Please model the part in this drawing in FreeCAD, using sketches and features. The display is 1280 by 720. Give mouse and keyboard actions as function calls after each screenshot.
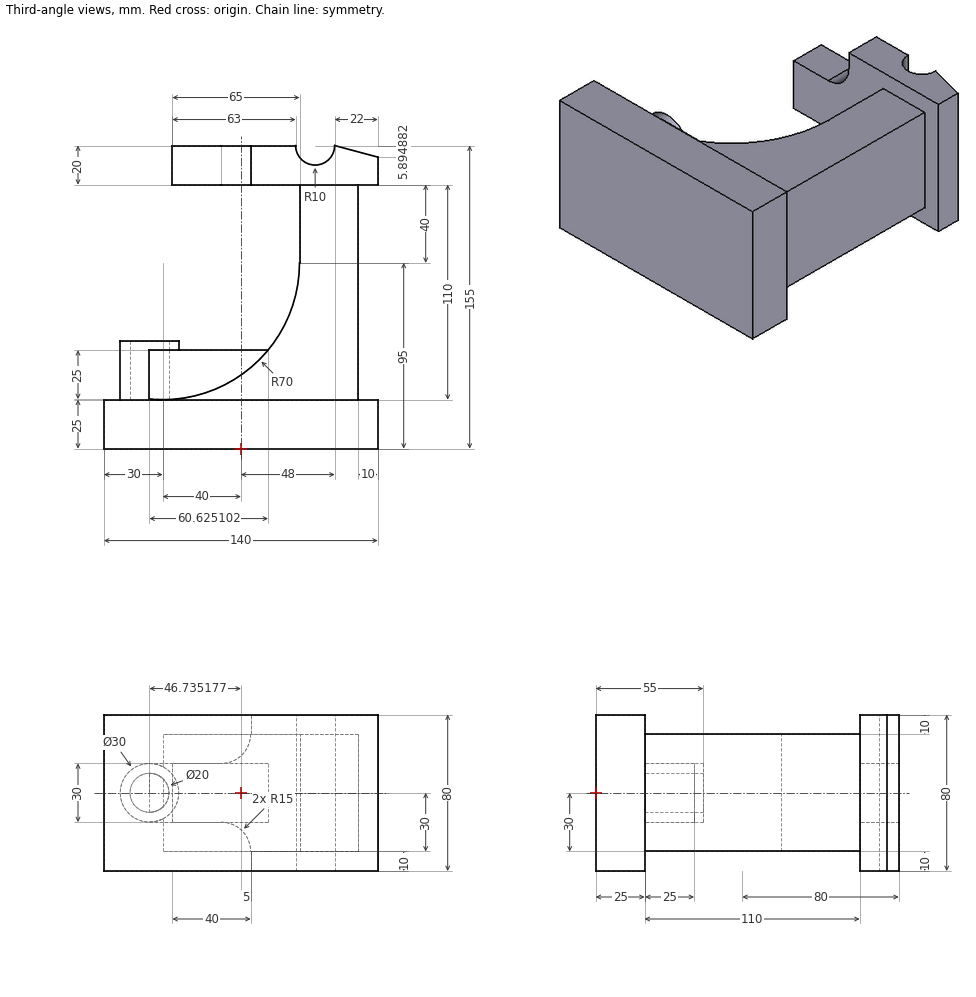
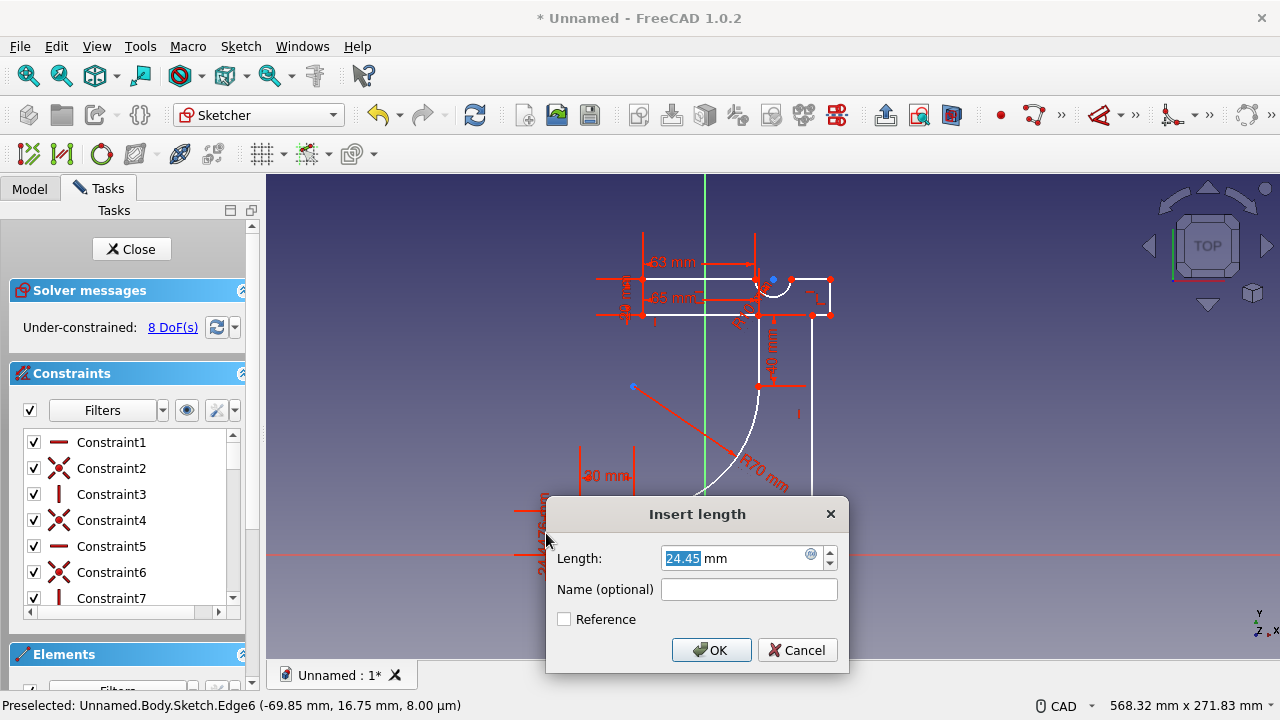
text(25)
key(Return)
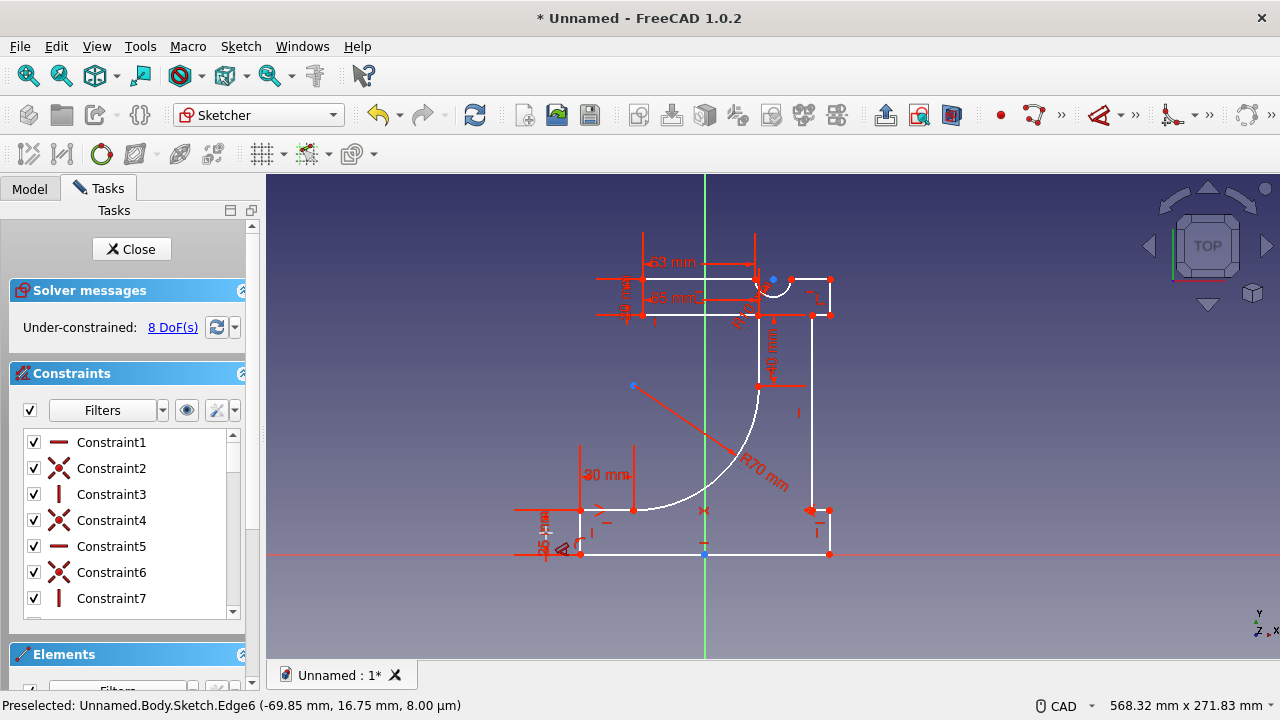
scroll(821, 510, up, 4)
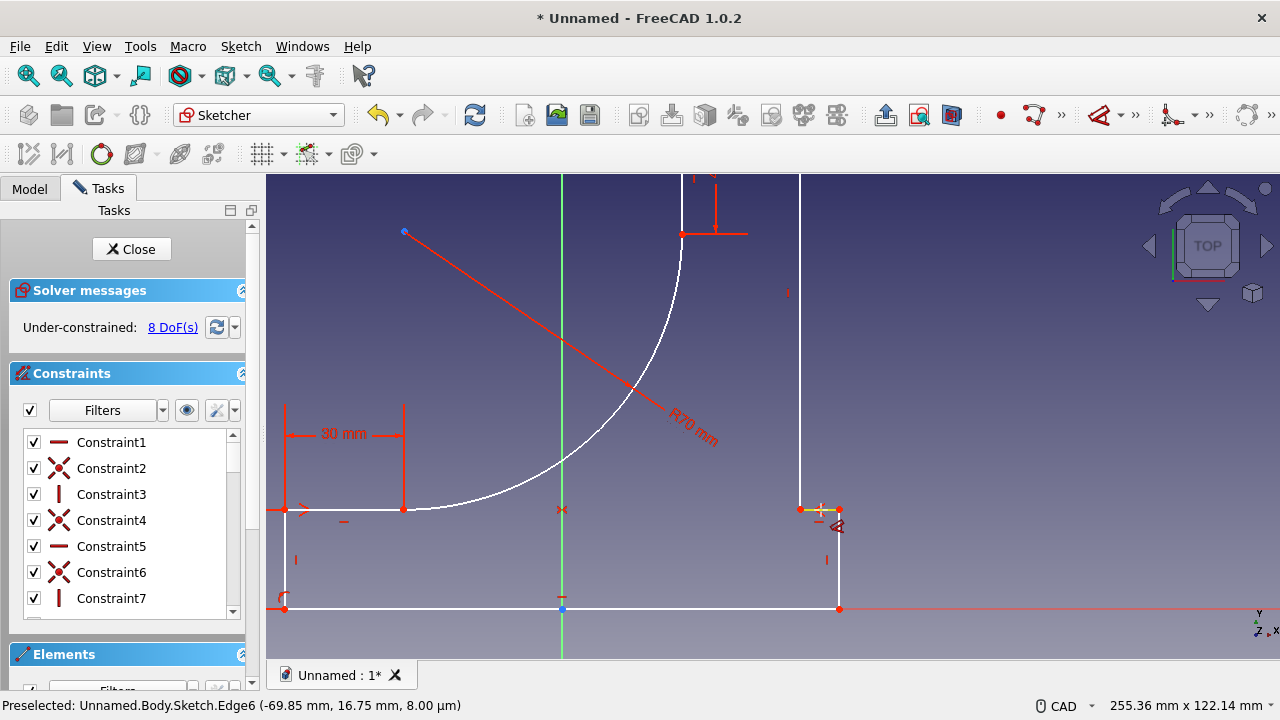
click(820, 510)
click(820, 544)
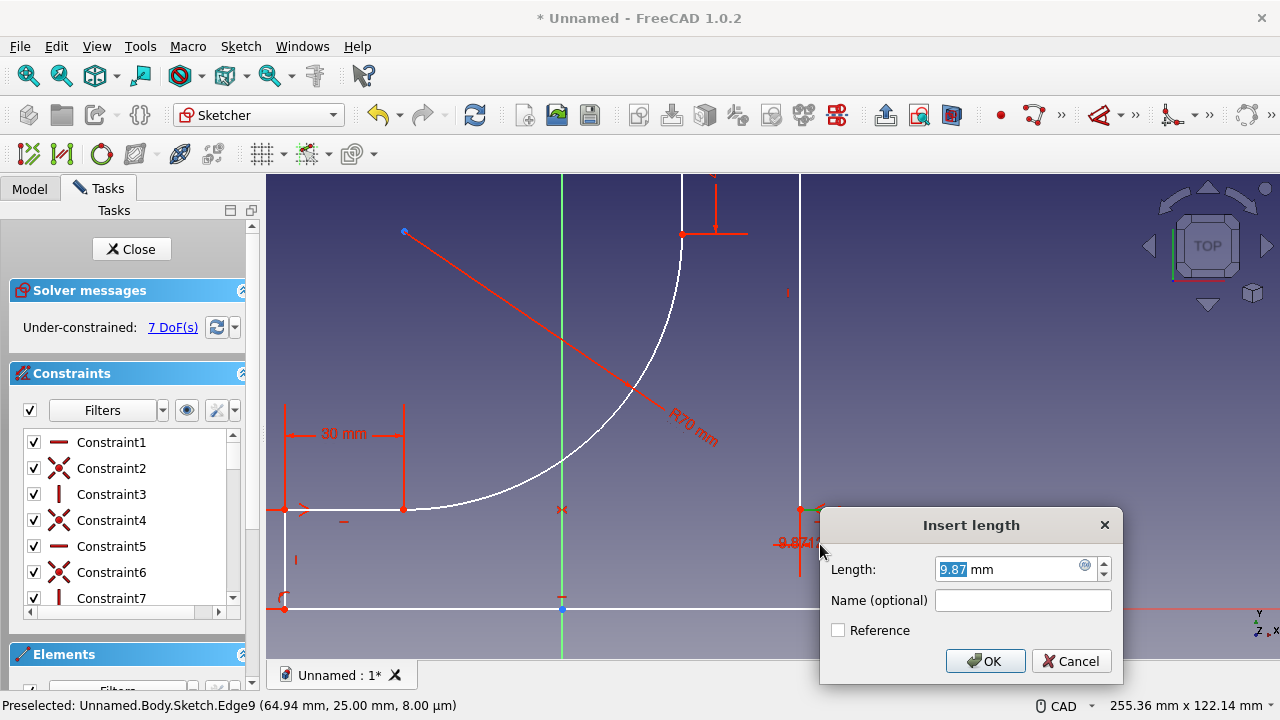
text(10)
key(Return)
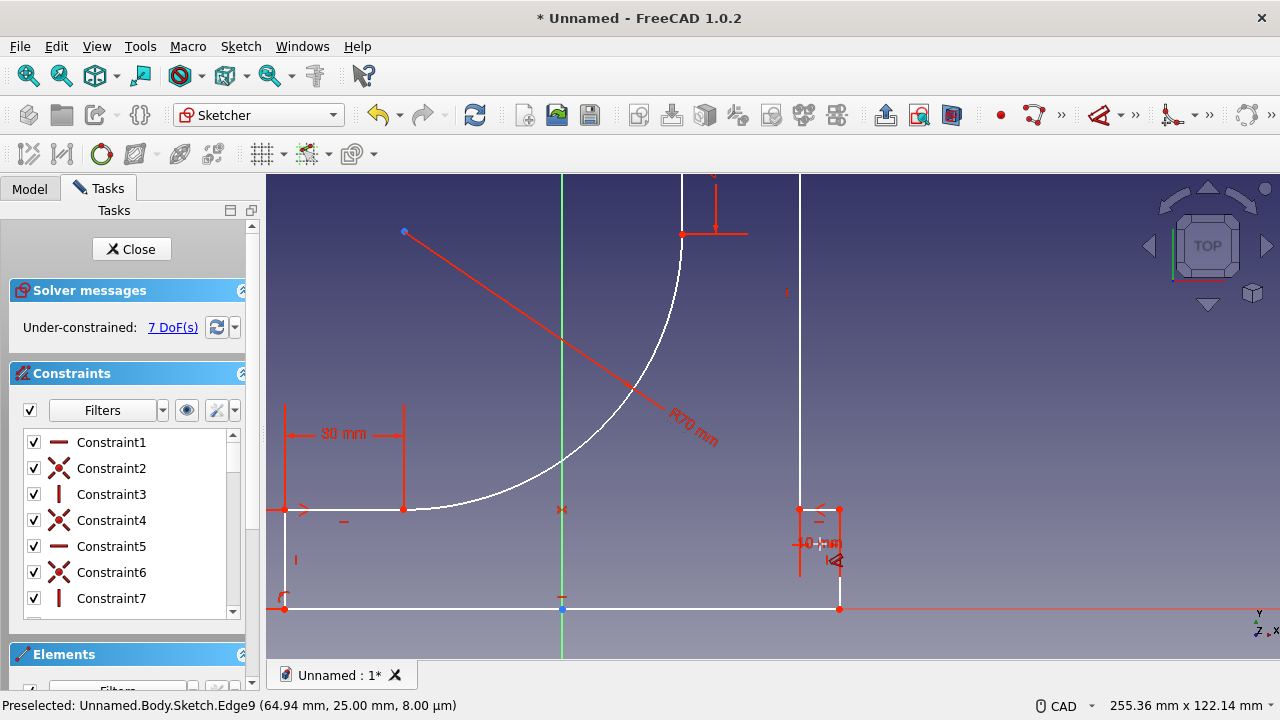
scroll(821, 510, down, 4)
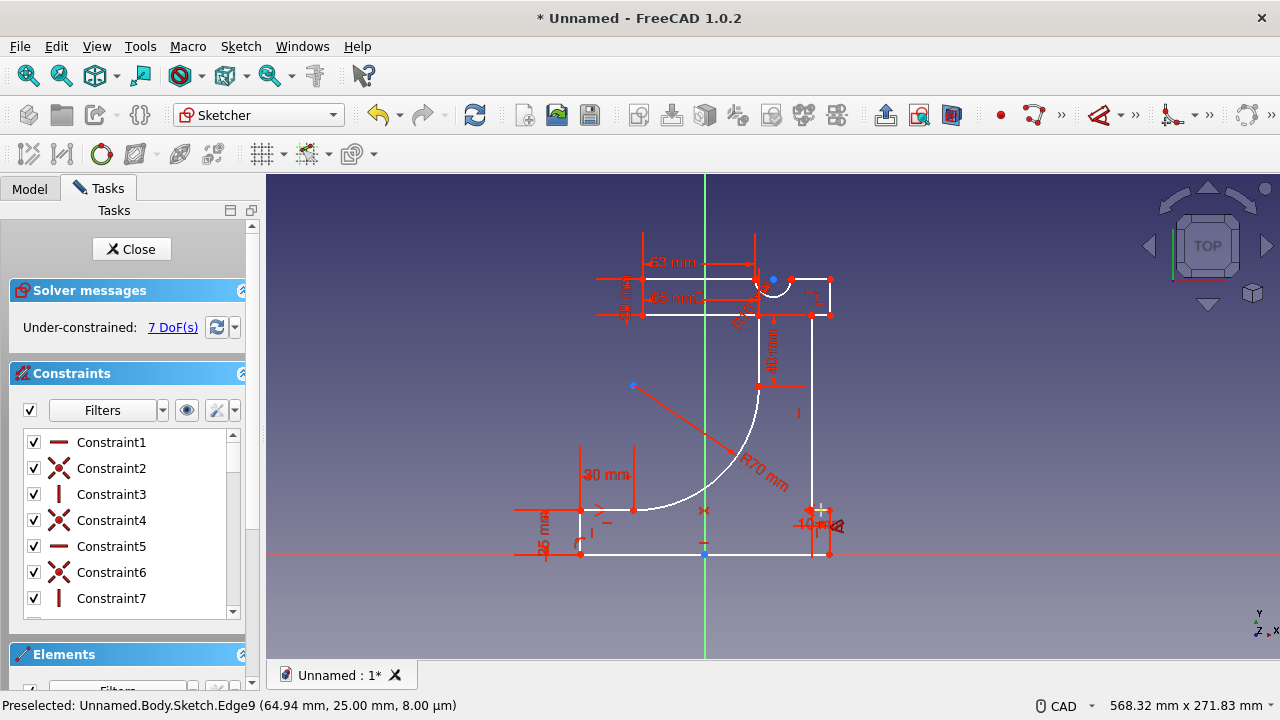
scroll(817, 315, up, 5)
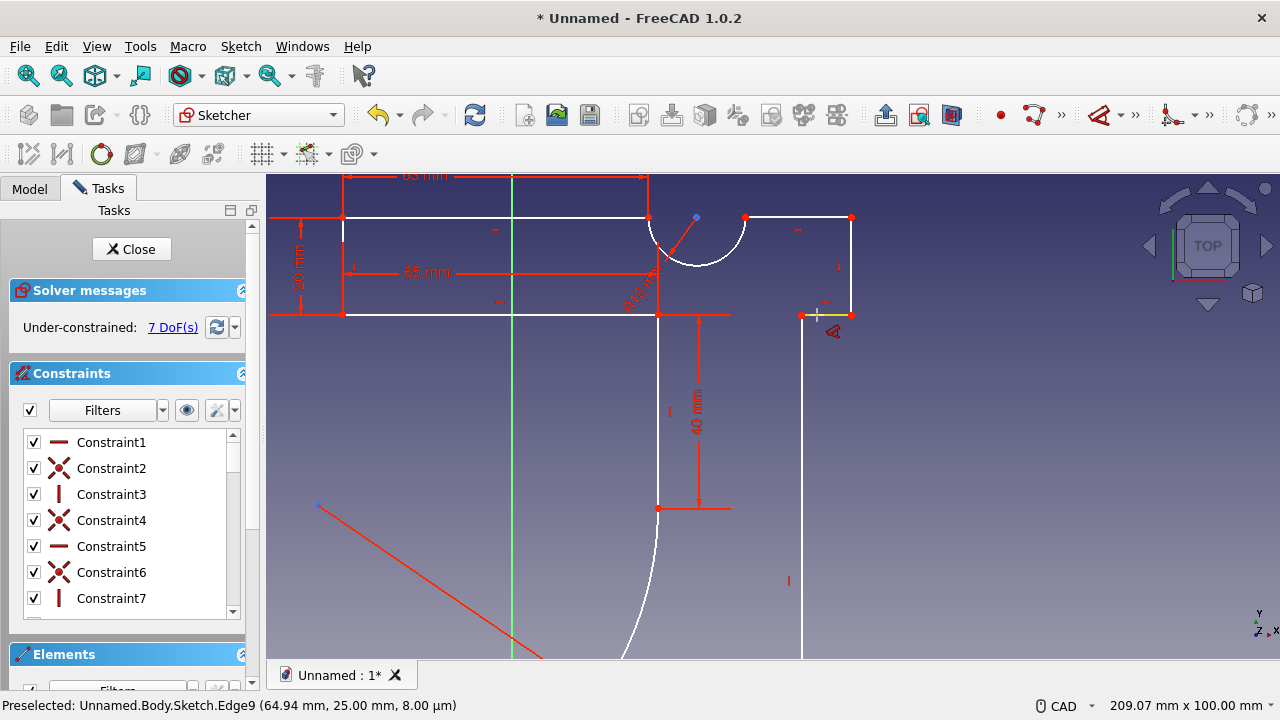
click(817, 315)
click(827, 281)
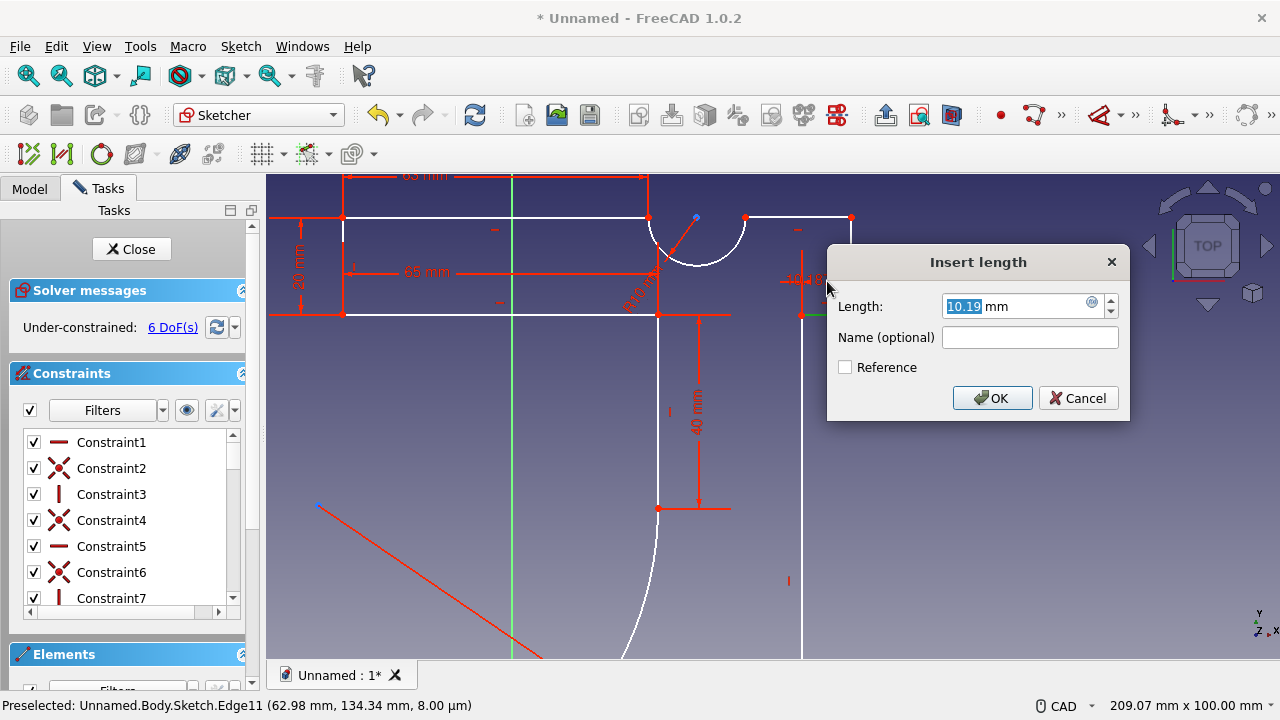
text(10)
key(Return)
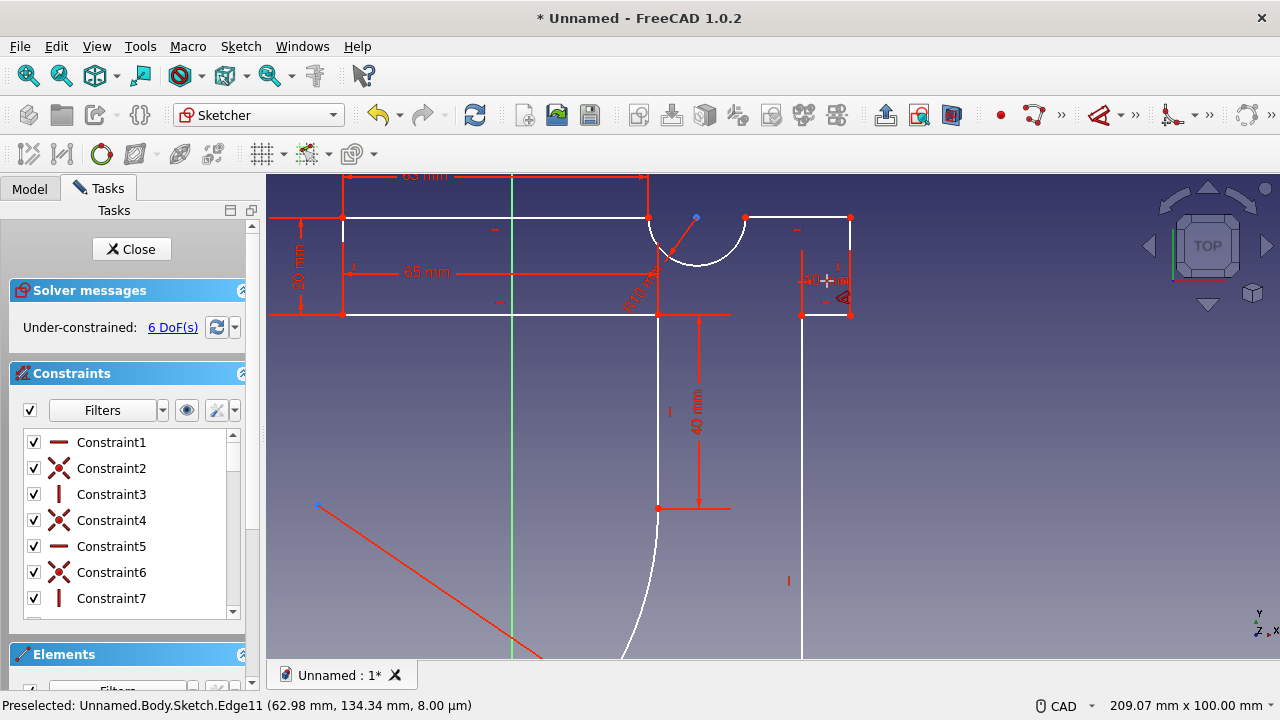
click(850, 286)
click(884, 244)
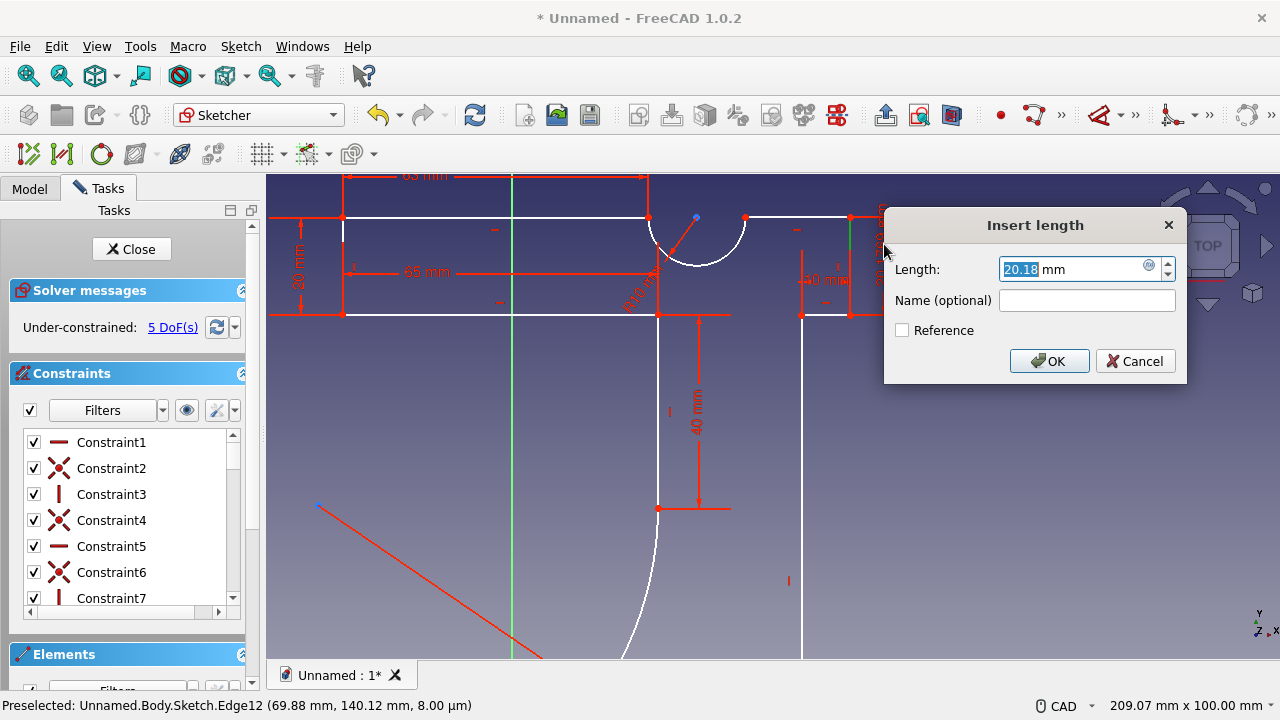
text(20)
key(Return)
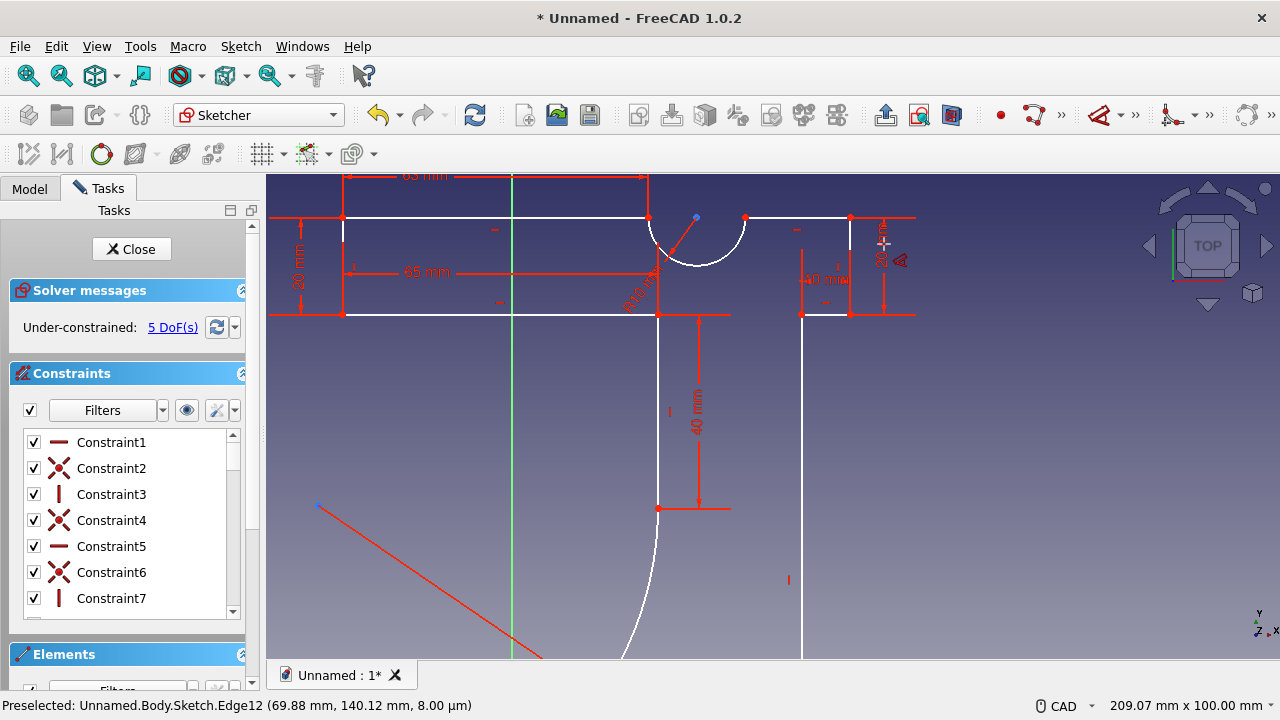
click(819, 218)
click(798, 252)